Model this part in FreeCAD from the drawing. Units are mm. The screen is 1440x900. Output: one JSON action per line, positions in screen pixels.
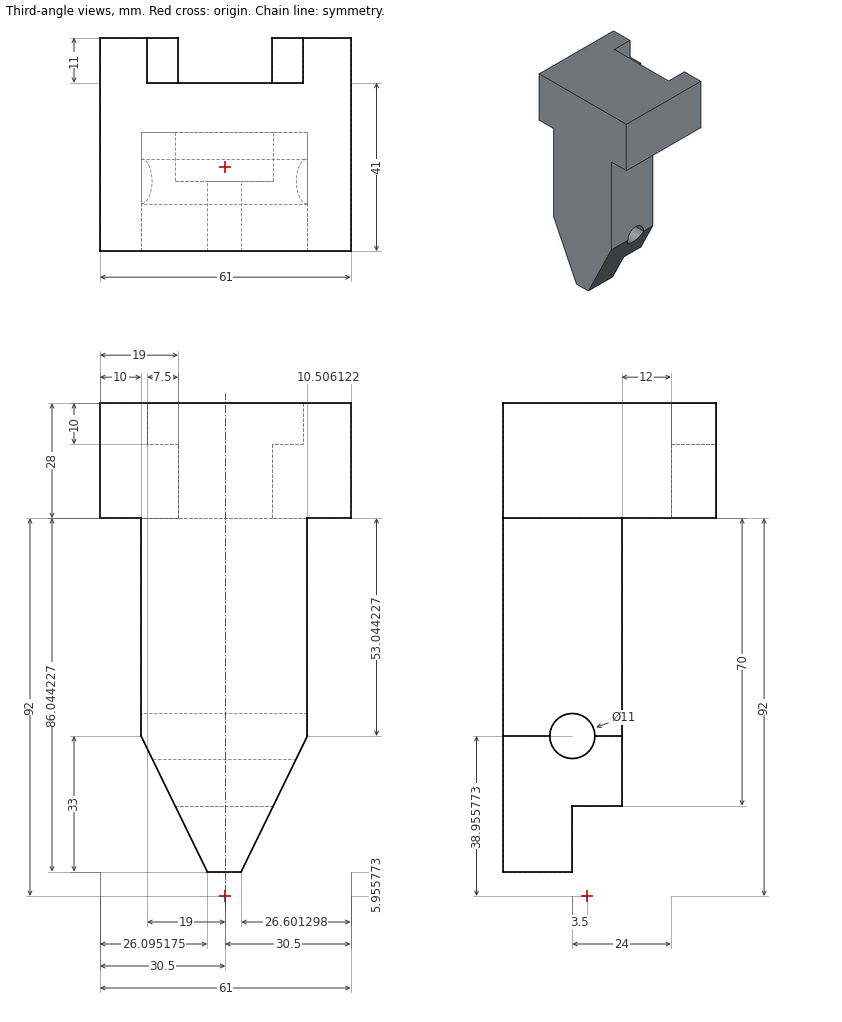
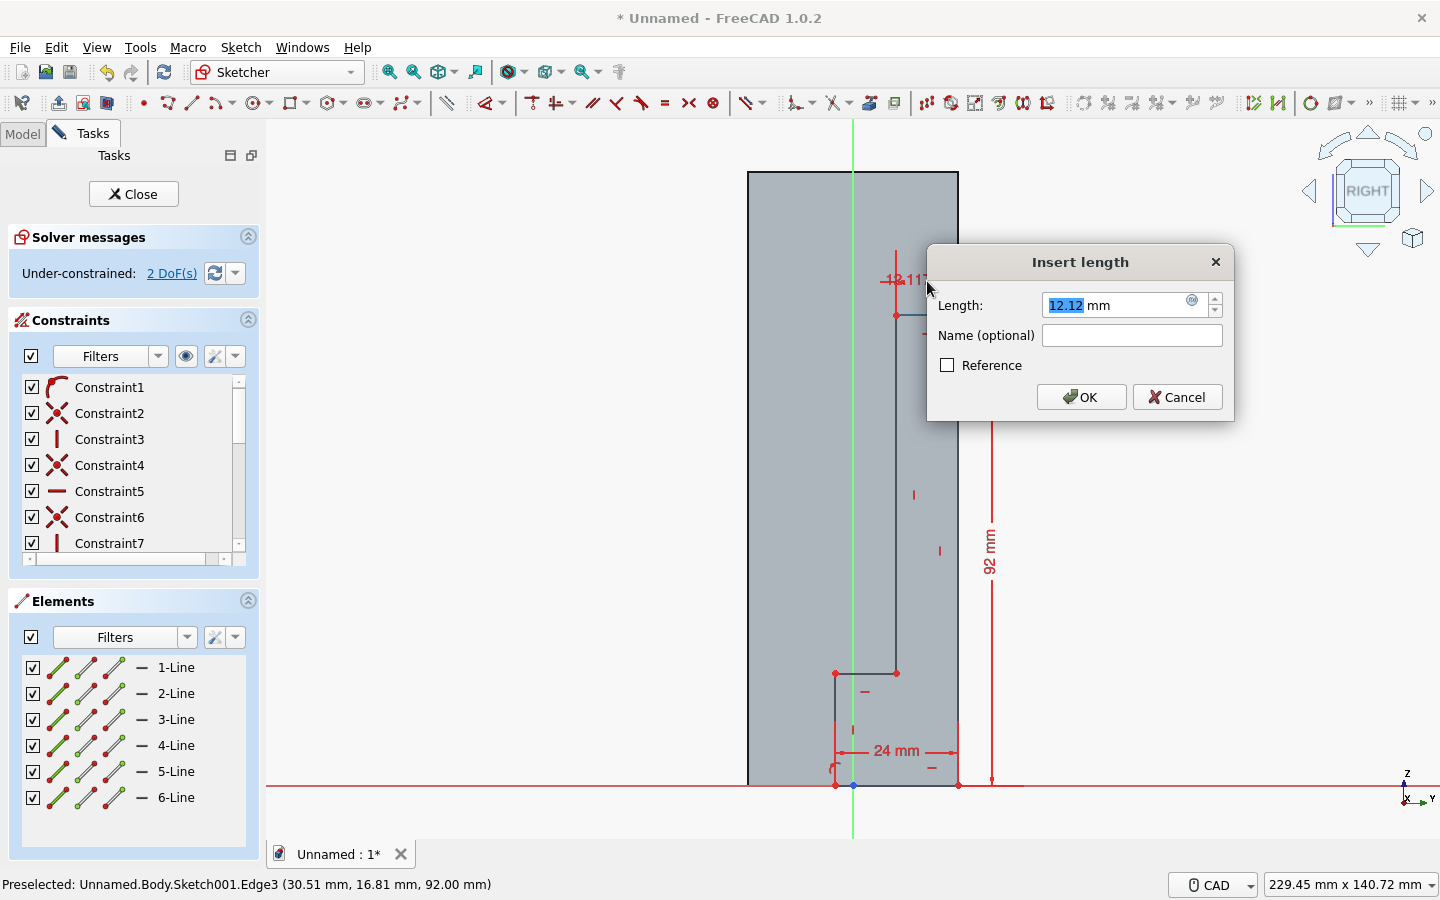
{"action": "type", "text": "12"}
{"action": "key", "text": "Return"}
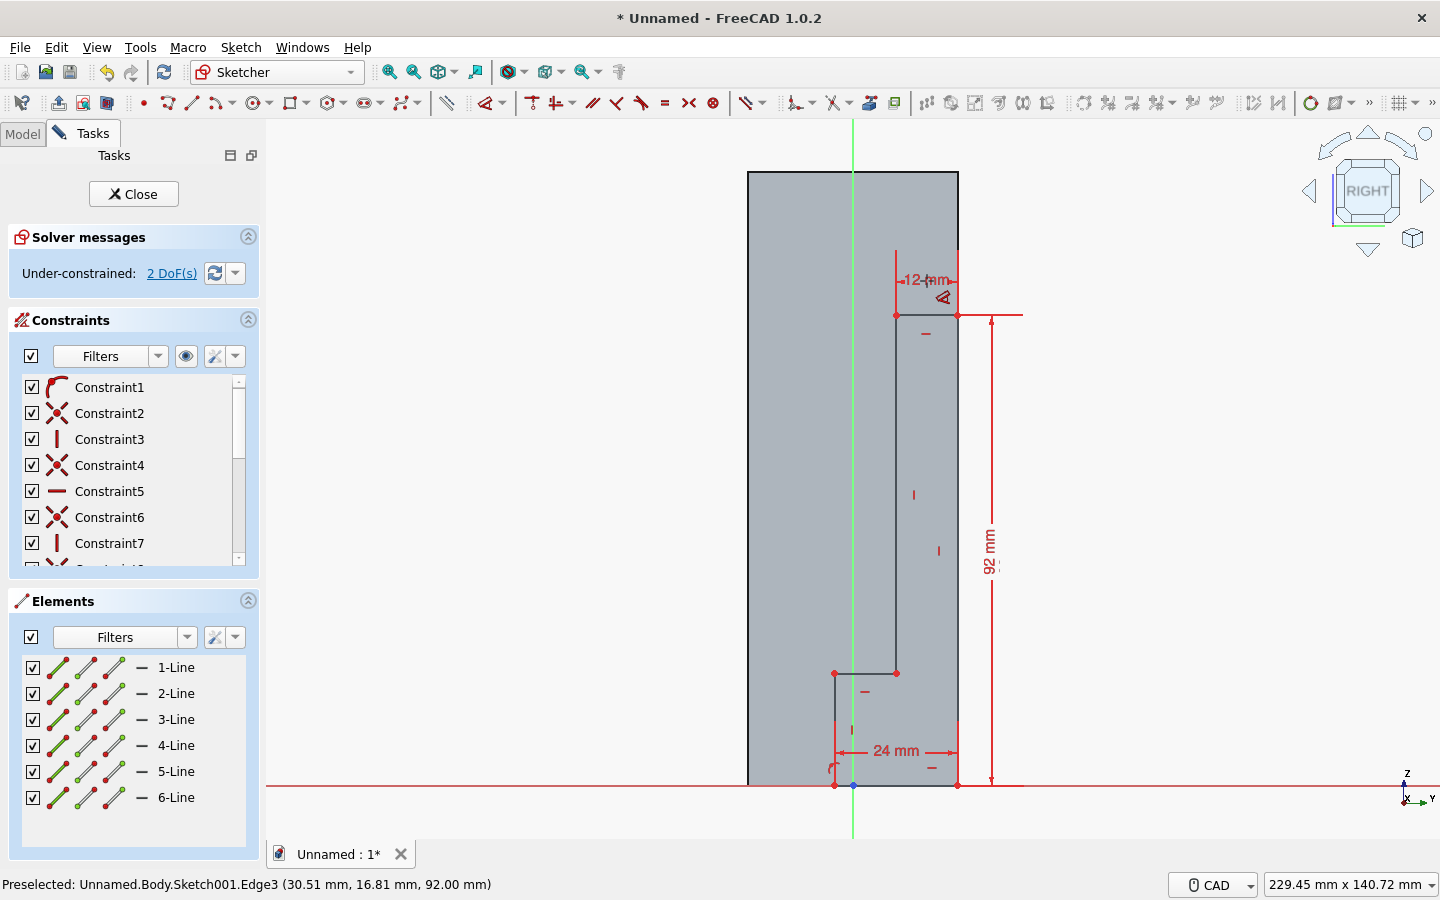
{"action": "left_click", "coordinate": [896, 423]}
{"action": "left_click", "coordinate": [930, 495]}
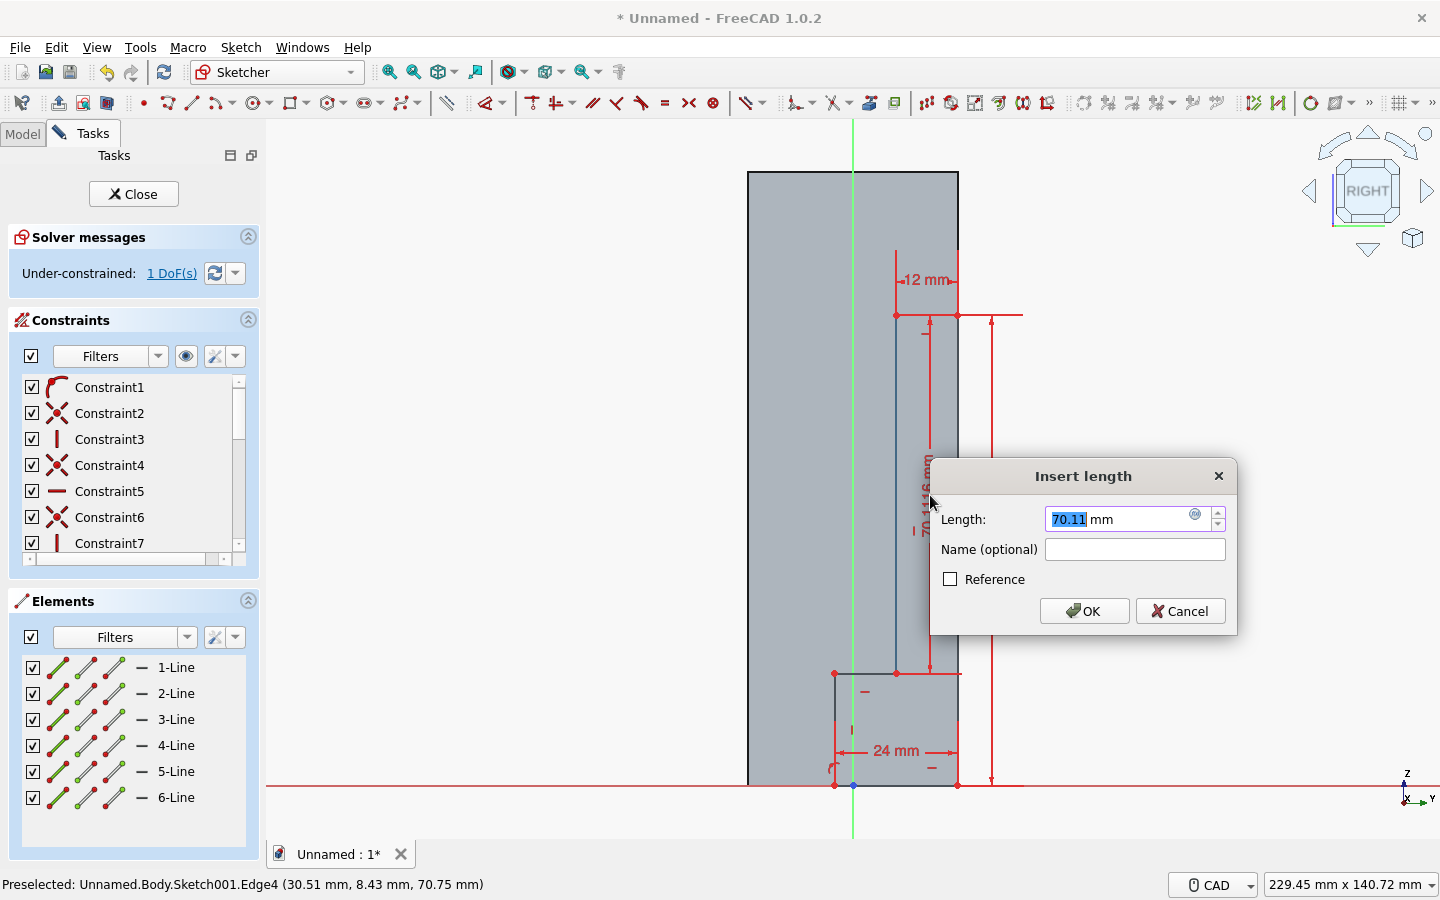
{"action": "type", "text": "70"}
{"action": "key", "text": "Return"}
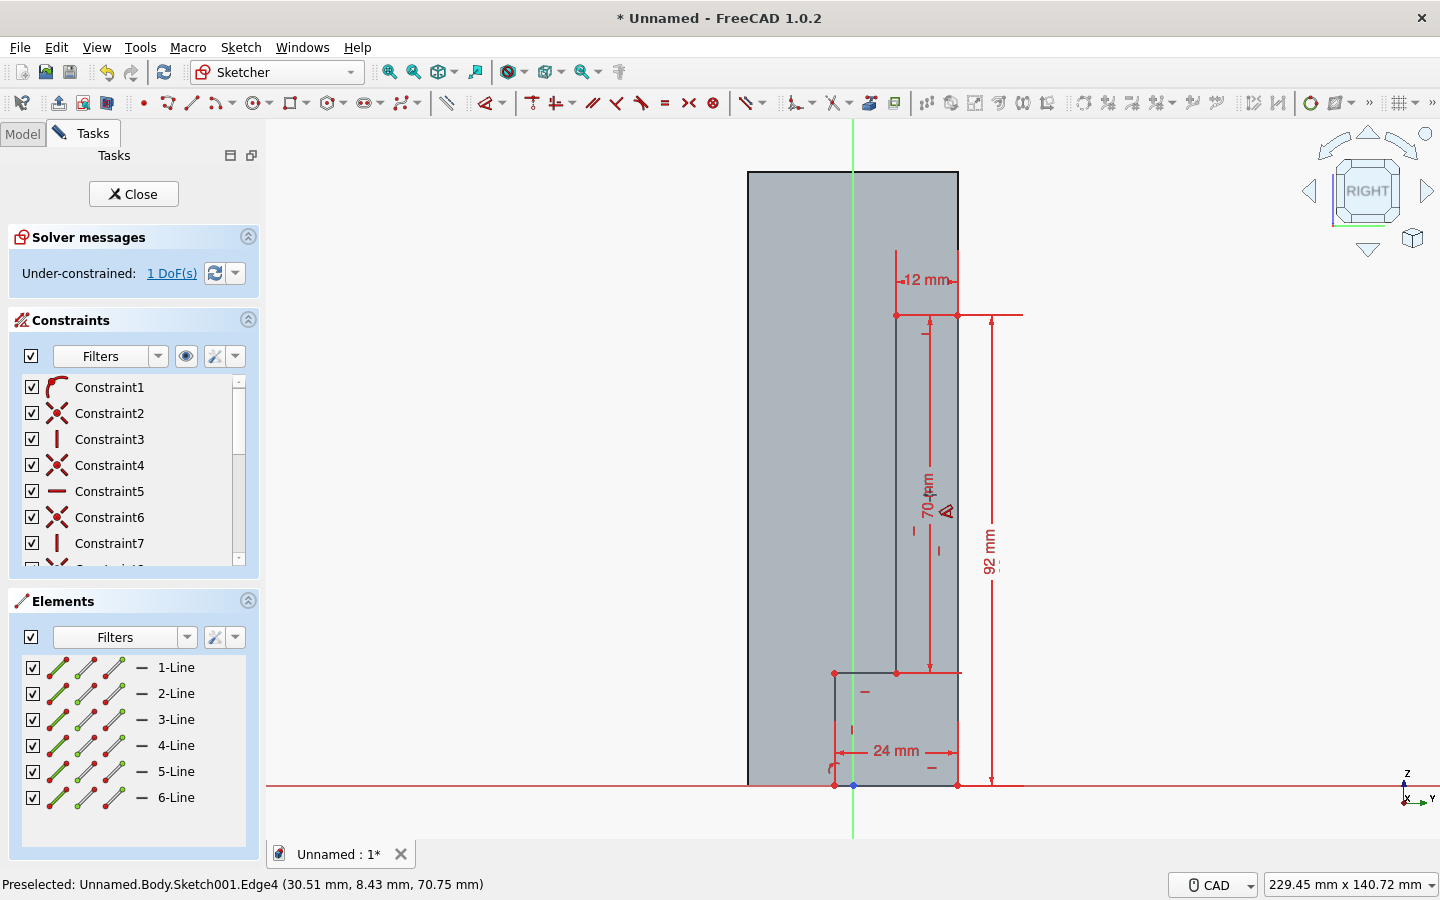
{"action": "scroll", "coordinate": [835, 786], "scroll_direction": "up", "scroll_amount": 4}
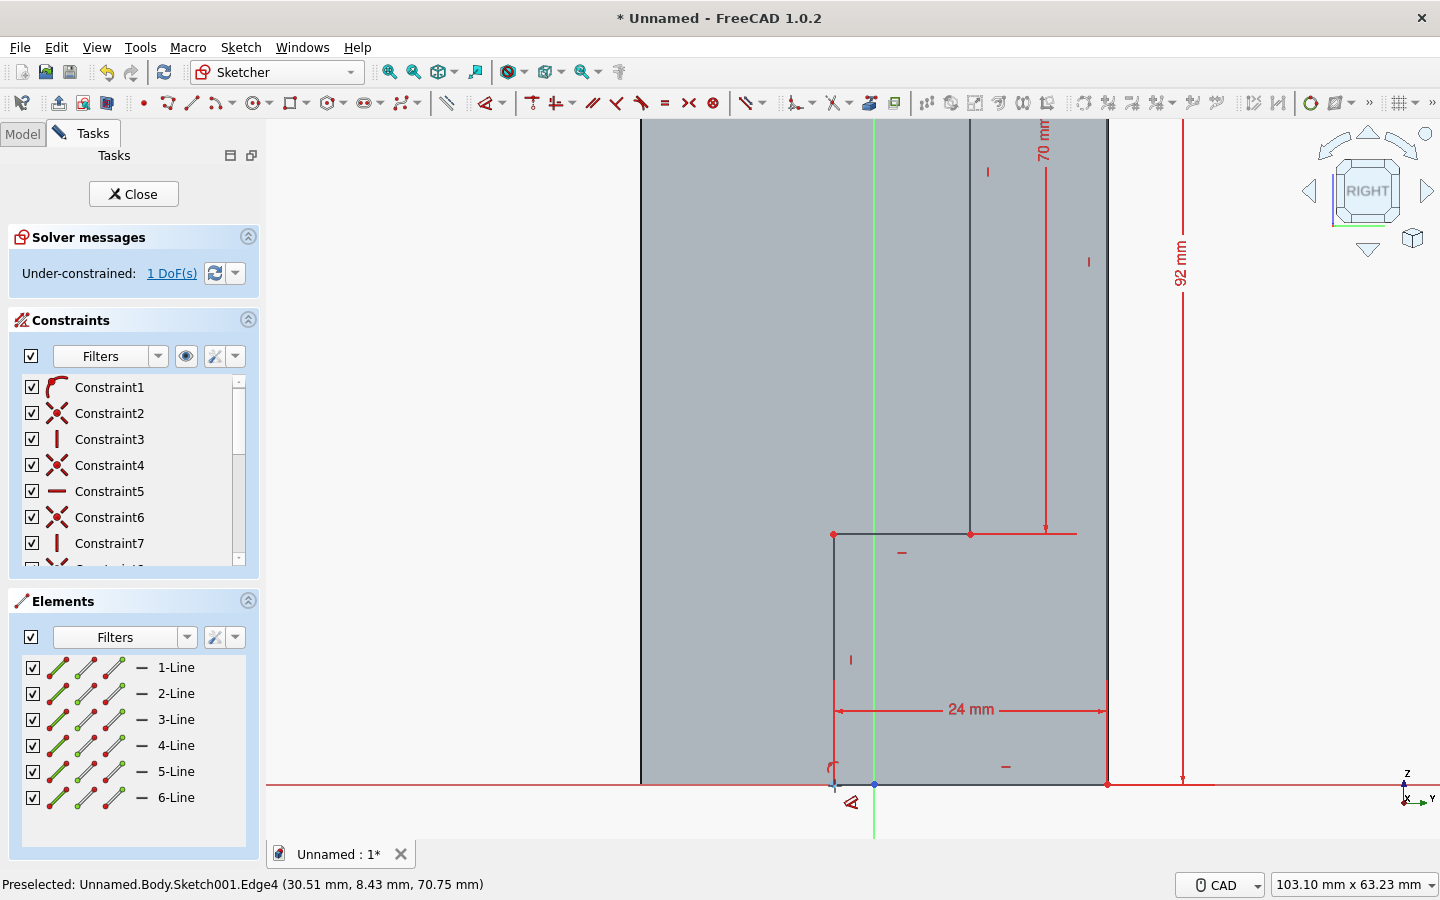
{"action": "left_click", "coordinate": [834, 785]}
{"action": "left_click", "coordinate": [854, 751]}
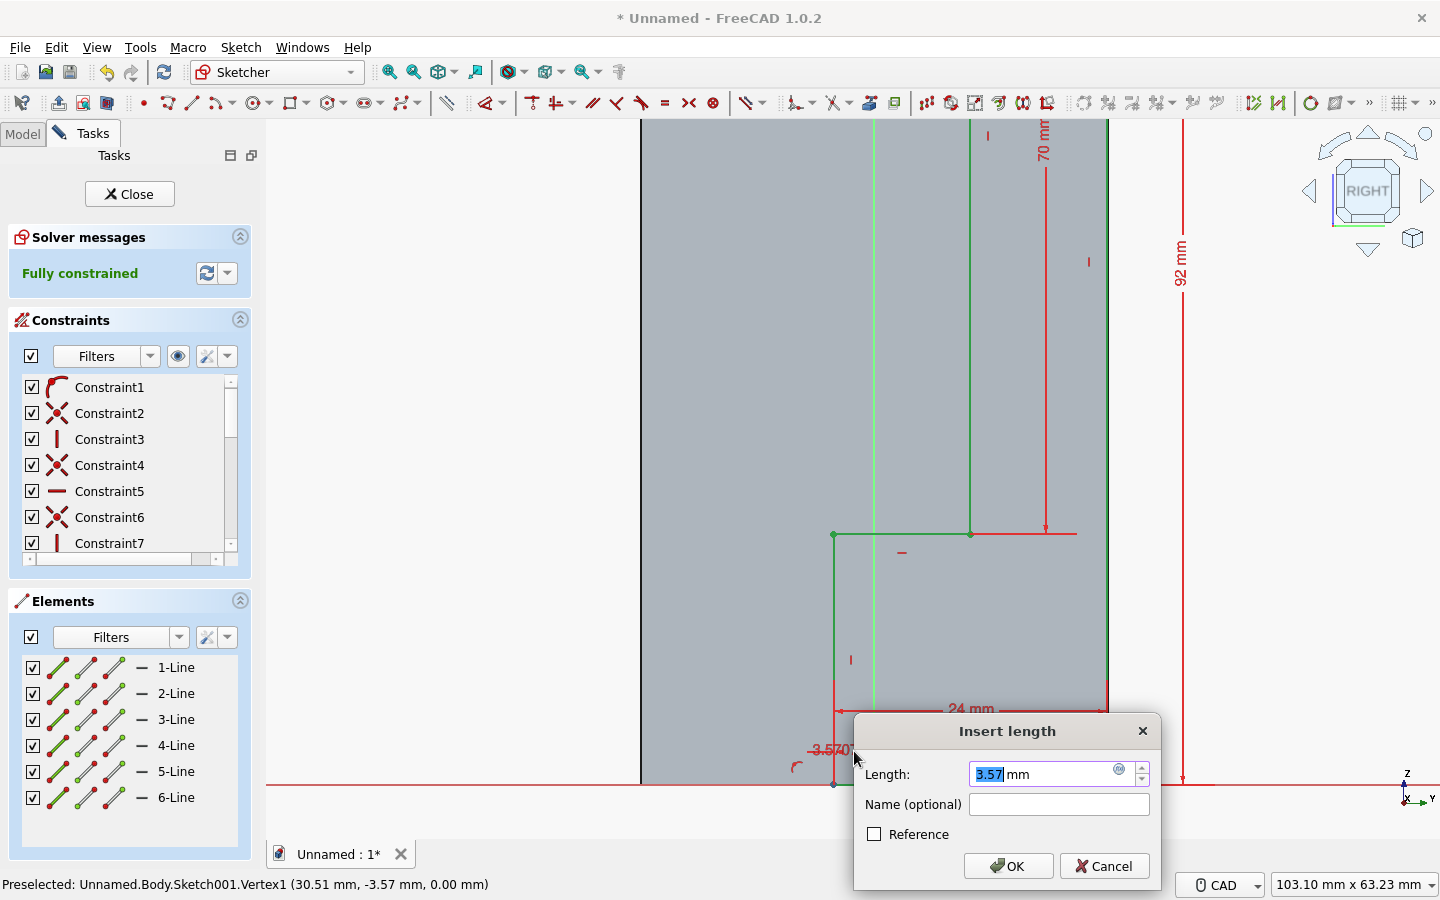
{"action": "type", "text": "3.5"}
{"action": "key", "text": "Return"}
{"action": "key", "text": "Escape"}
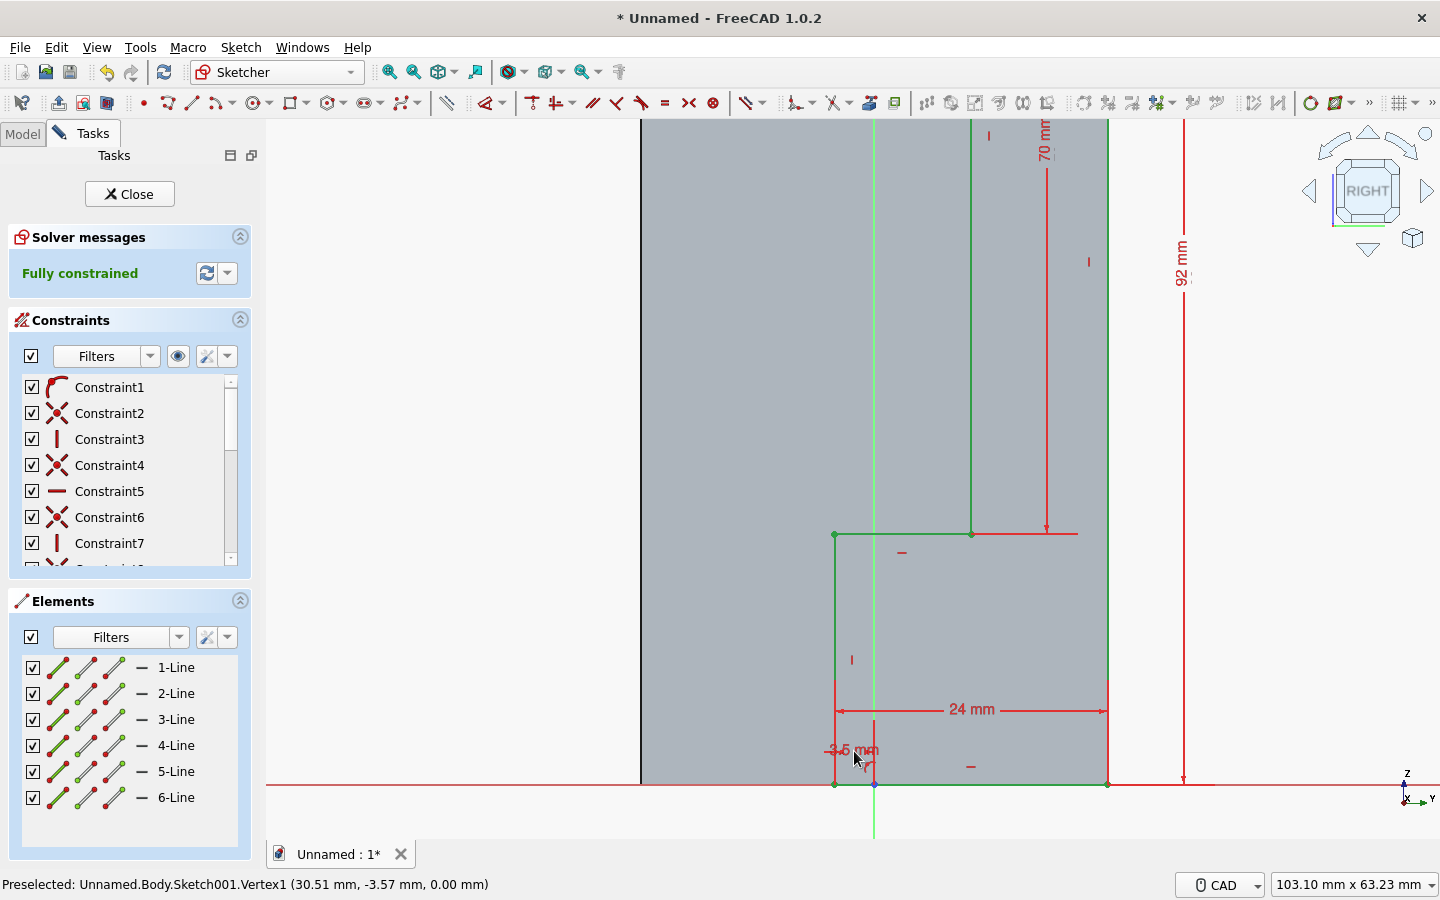
{"action": "left_click", "coordinate": [130, 194]}